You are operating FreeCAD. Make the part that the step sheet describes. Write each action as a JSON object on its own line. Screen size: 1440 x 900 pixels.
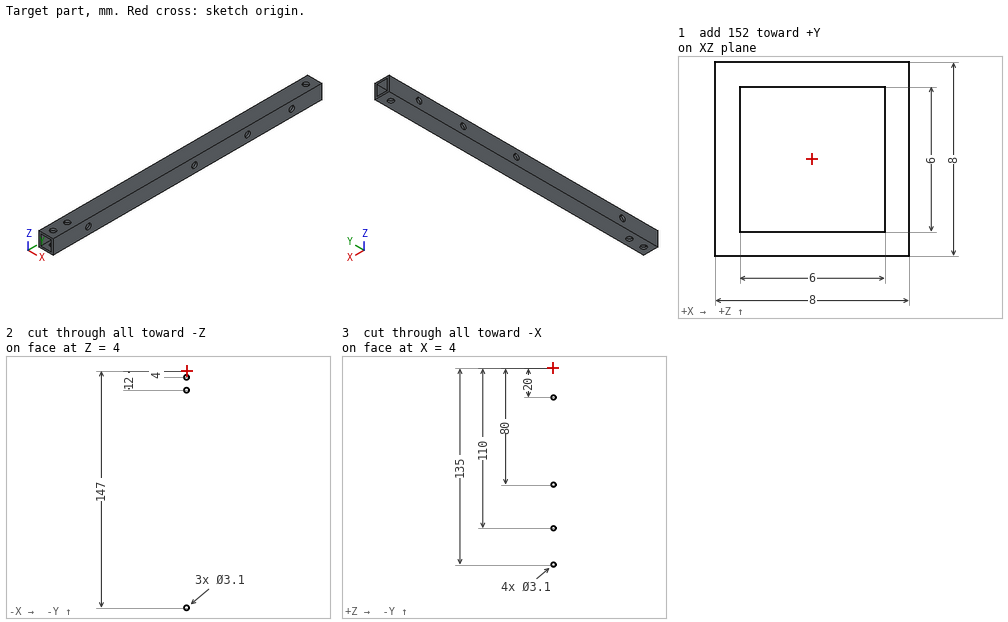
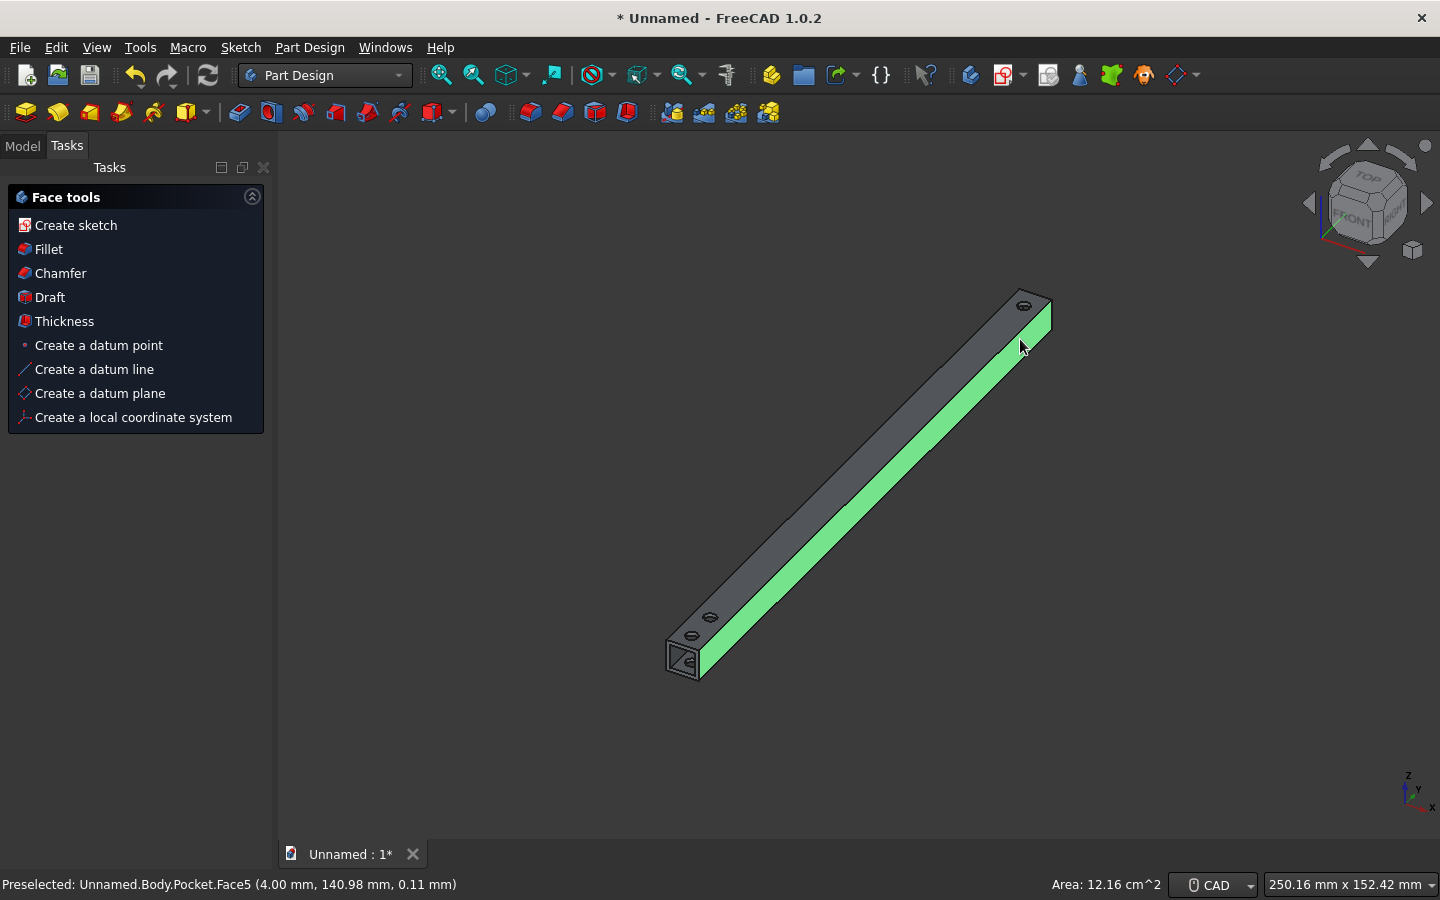
{"action": "left_click", "coordinate": [1004, 76]}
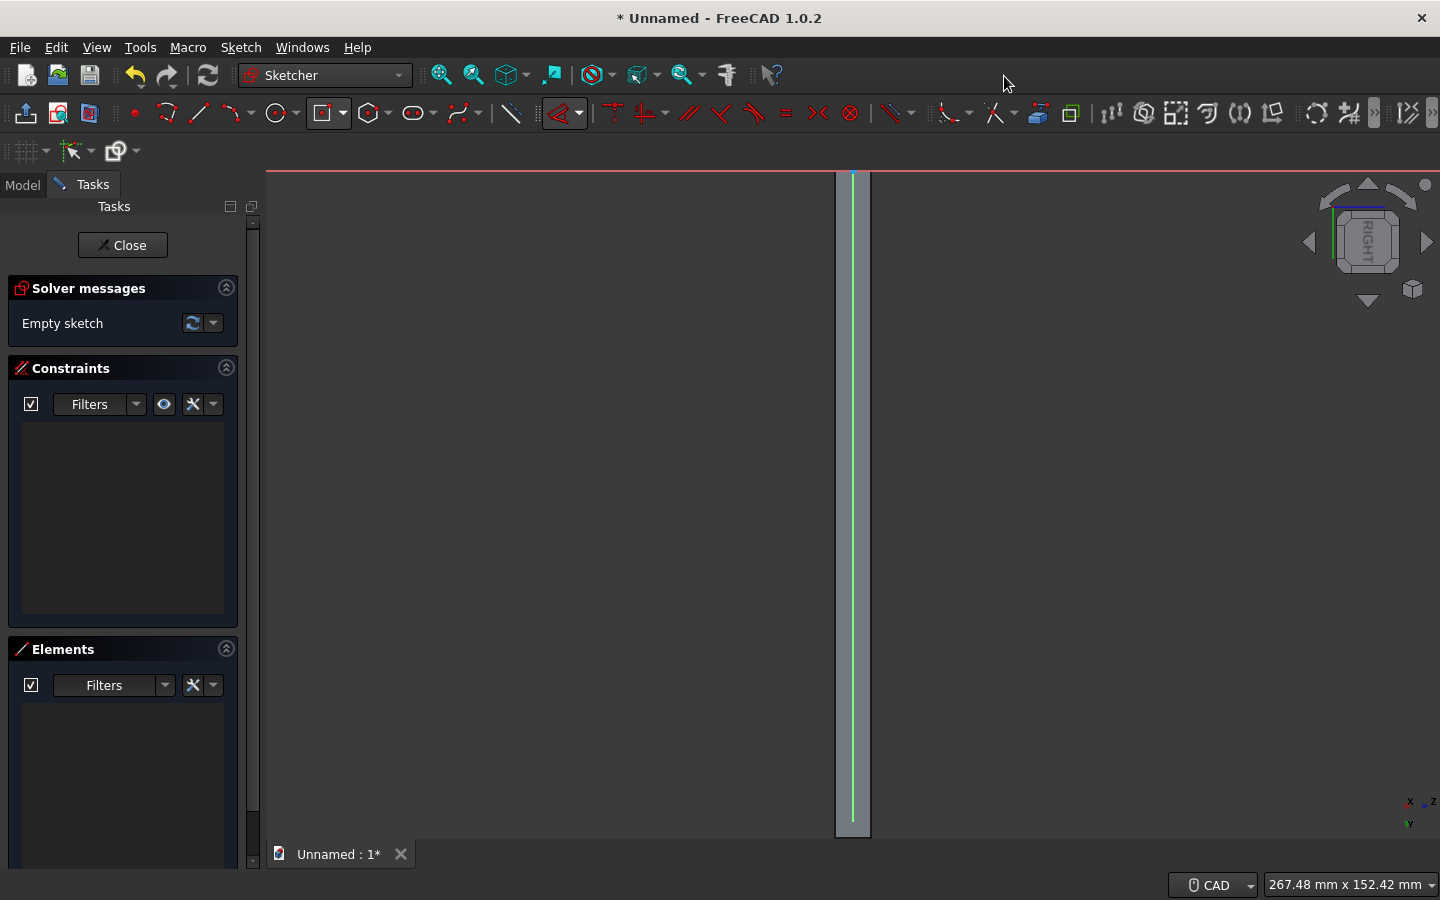
{"action": "scroll", "coordinate": [645, 573], "scroll_direction": "down", "scroll_amount": 2}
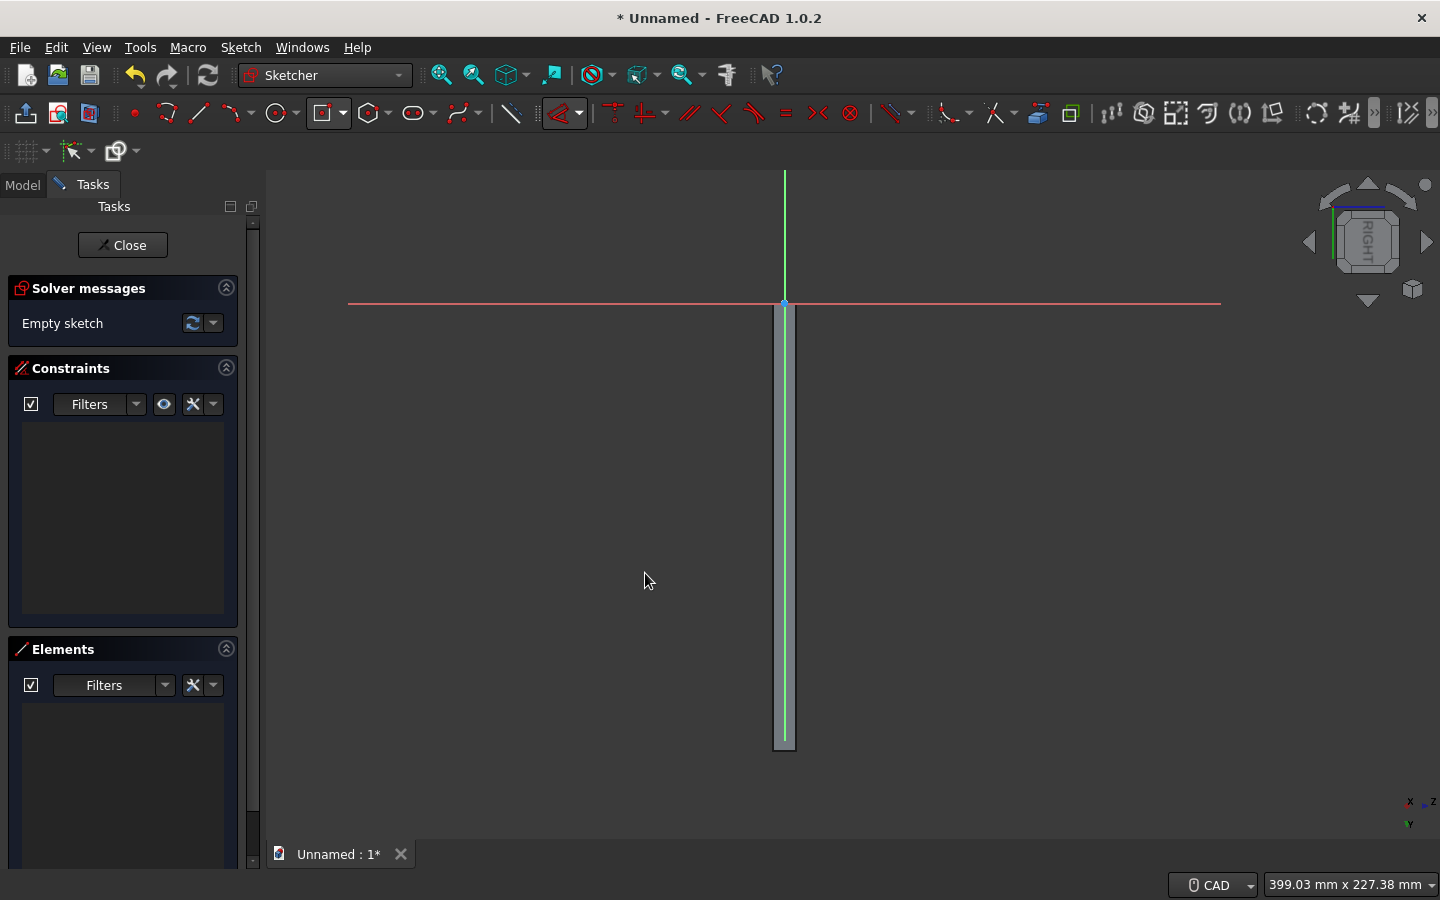
{"action": "key", "text": "g c"}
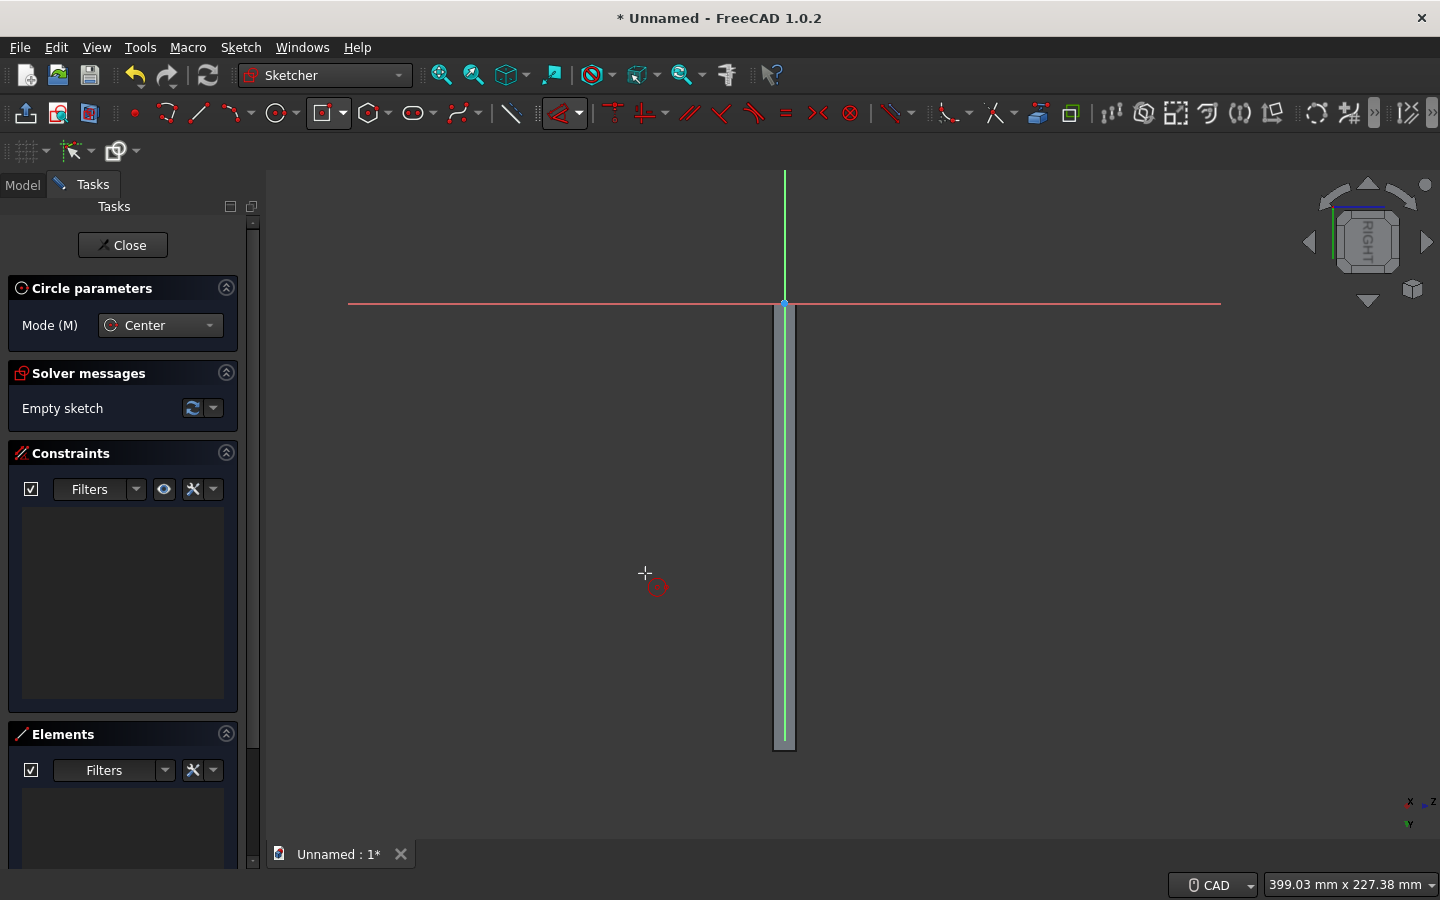
{"action": "scroll", "coordinate": [785, 701], "scroll_direction": "up", "scroll_amount": 9}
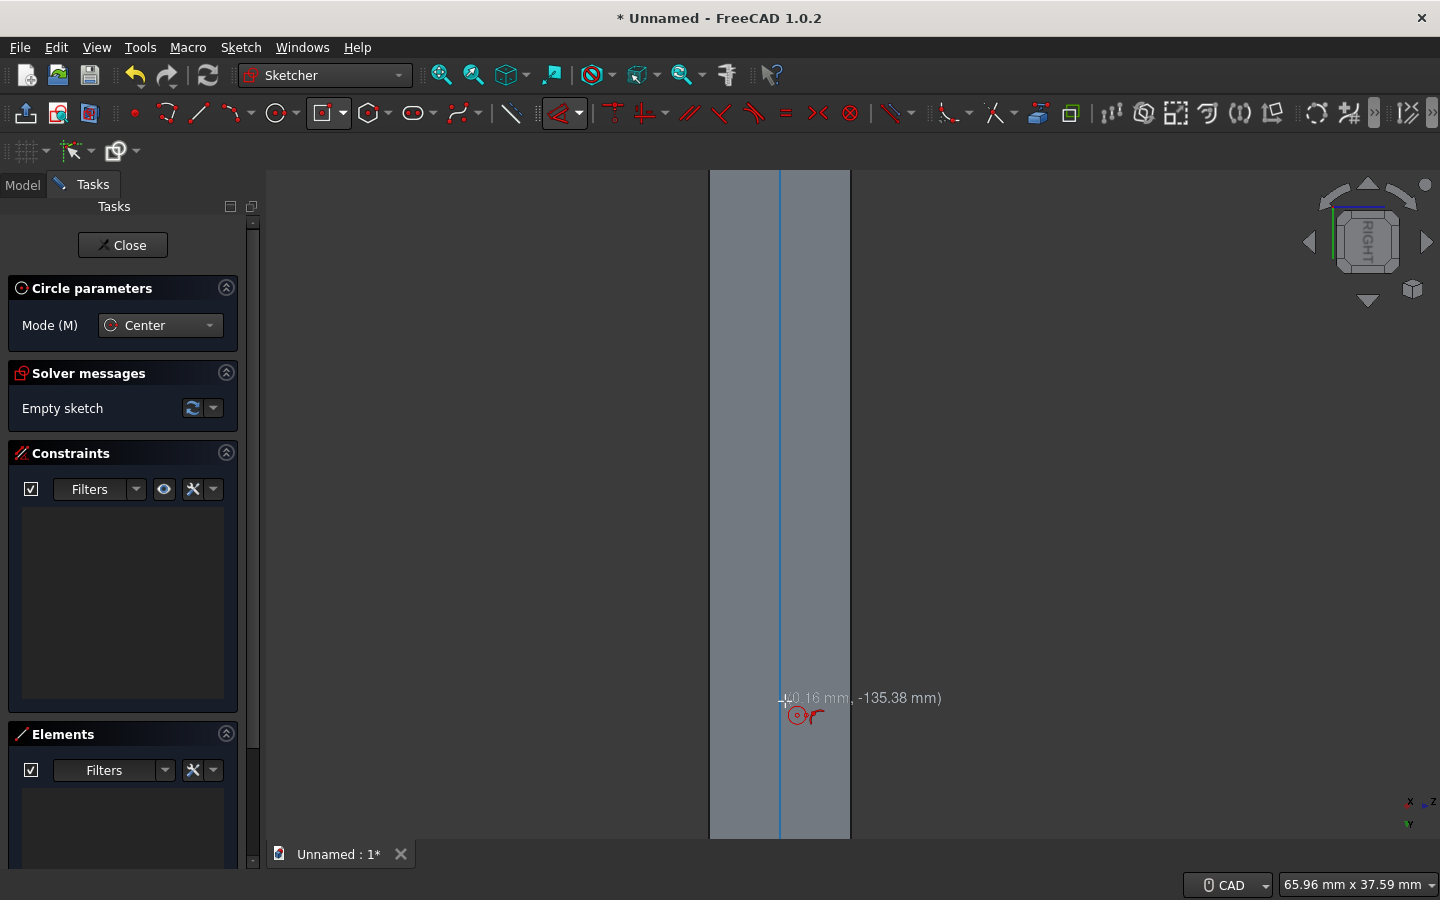
{"action": "scroll", "coordinate": [785, 702], "scroll_direction": "down", "scroll_amount": 9}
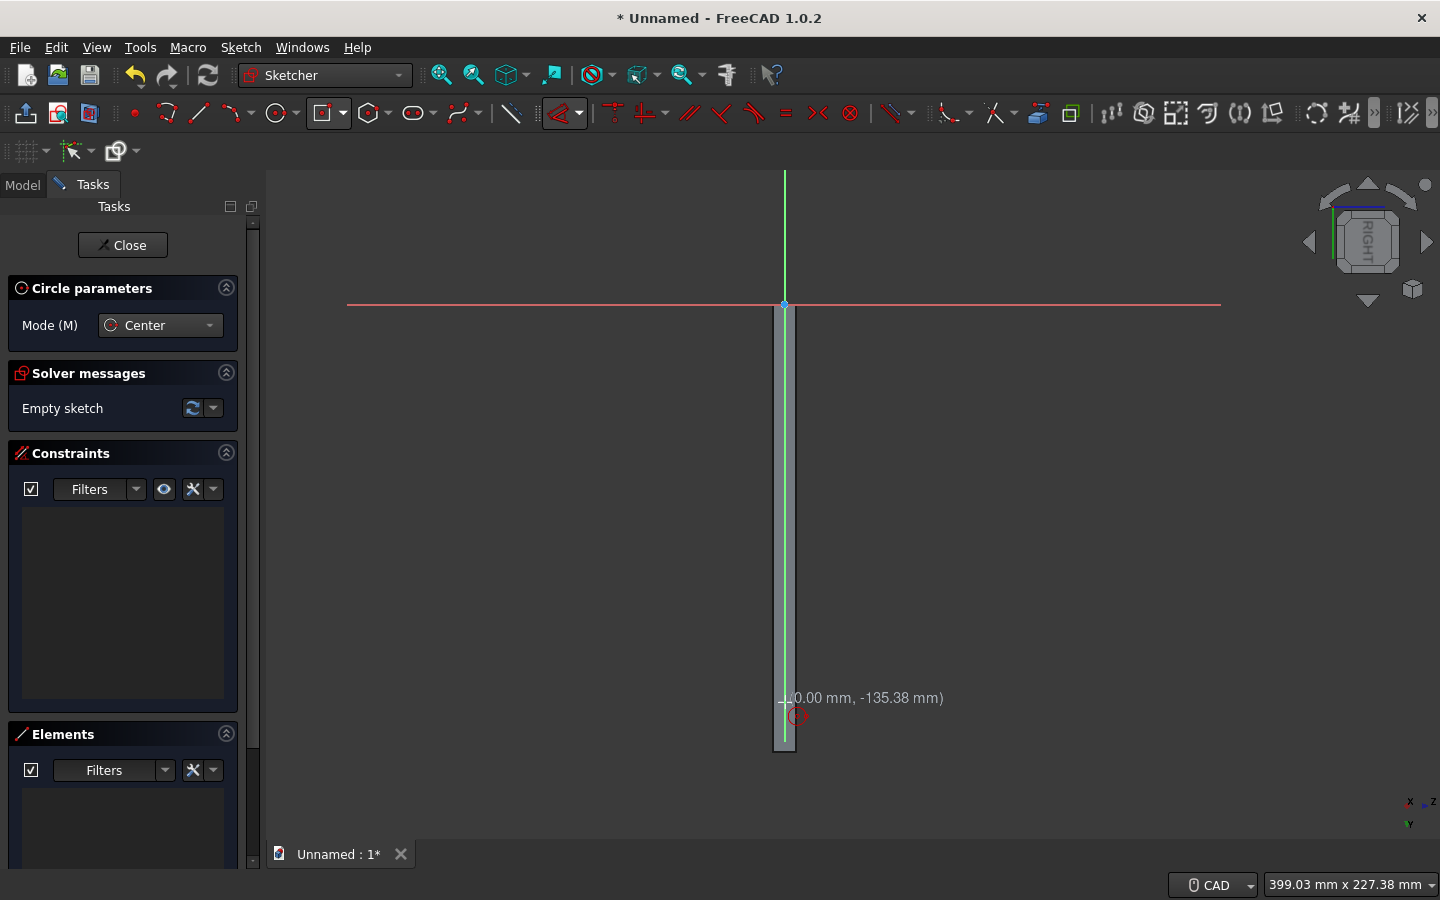
{"action": "left_click", "coordinate": [785, 702]}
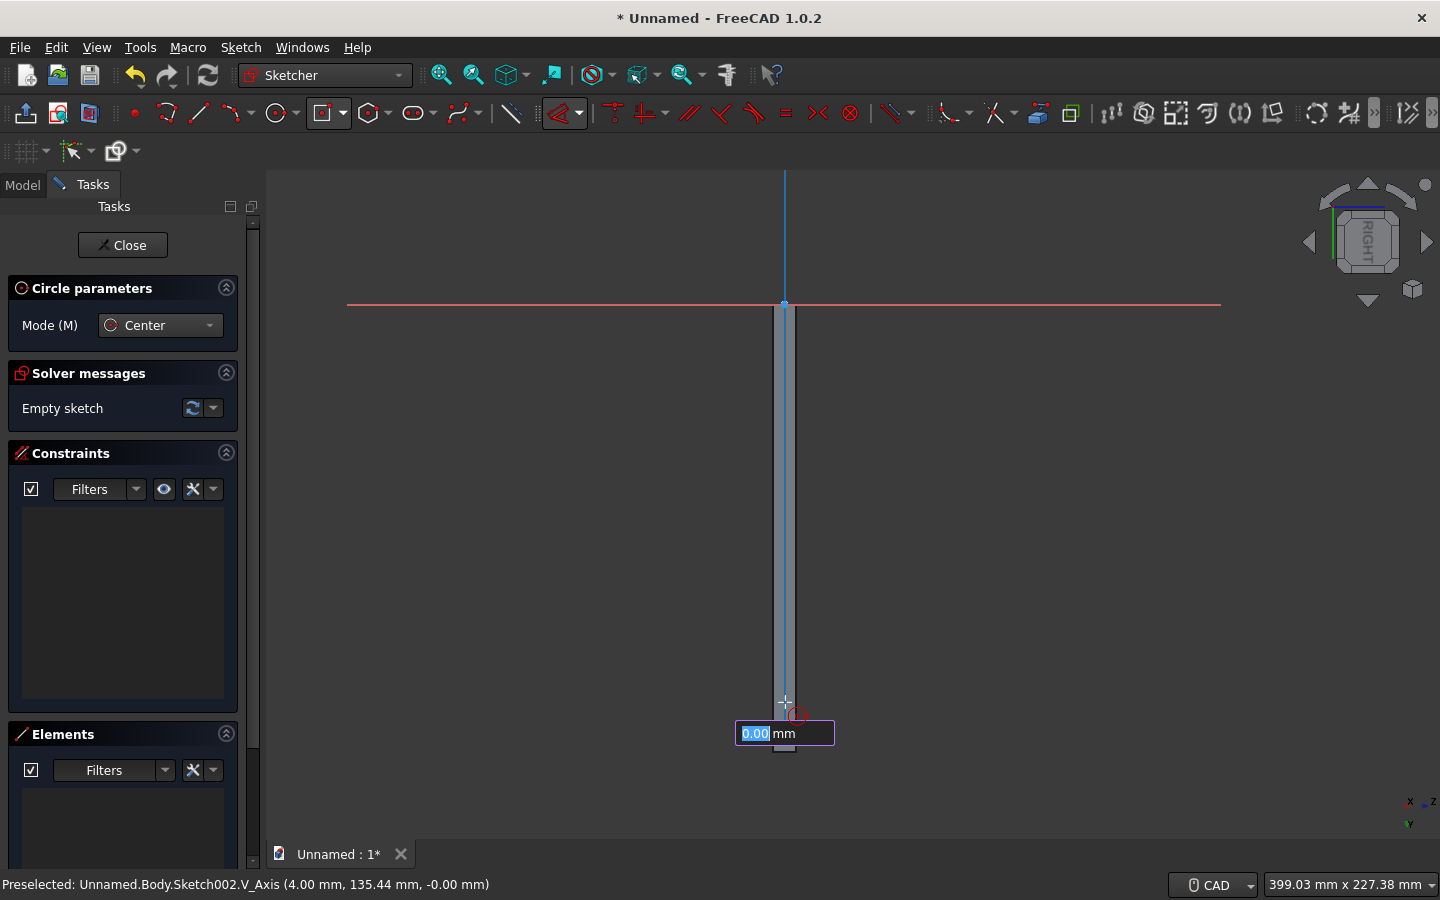
{"action": "scroll", "coordinate": [789, 700], "scroll_direction": "up", "scroll_amount": 7}
{"action": "mouse_move", "coordinate": [787, 698]}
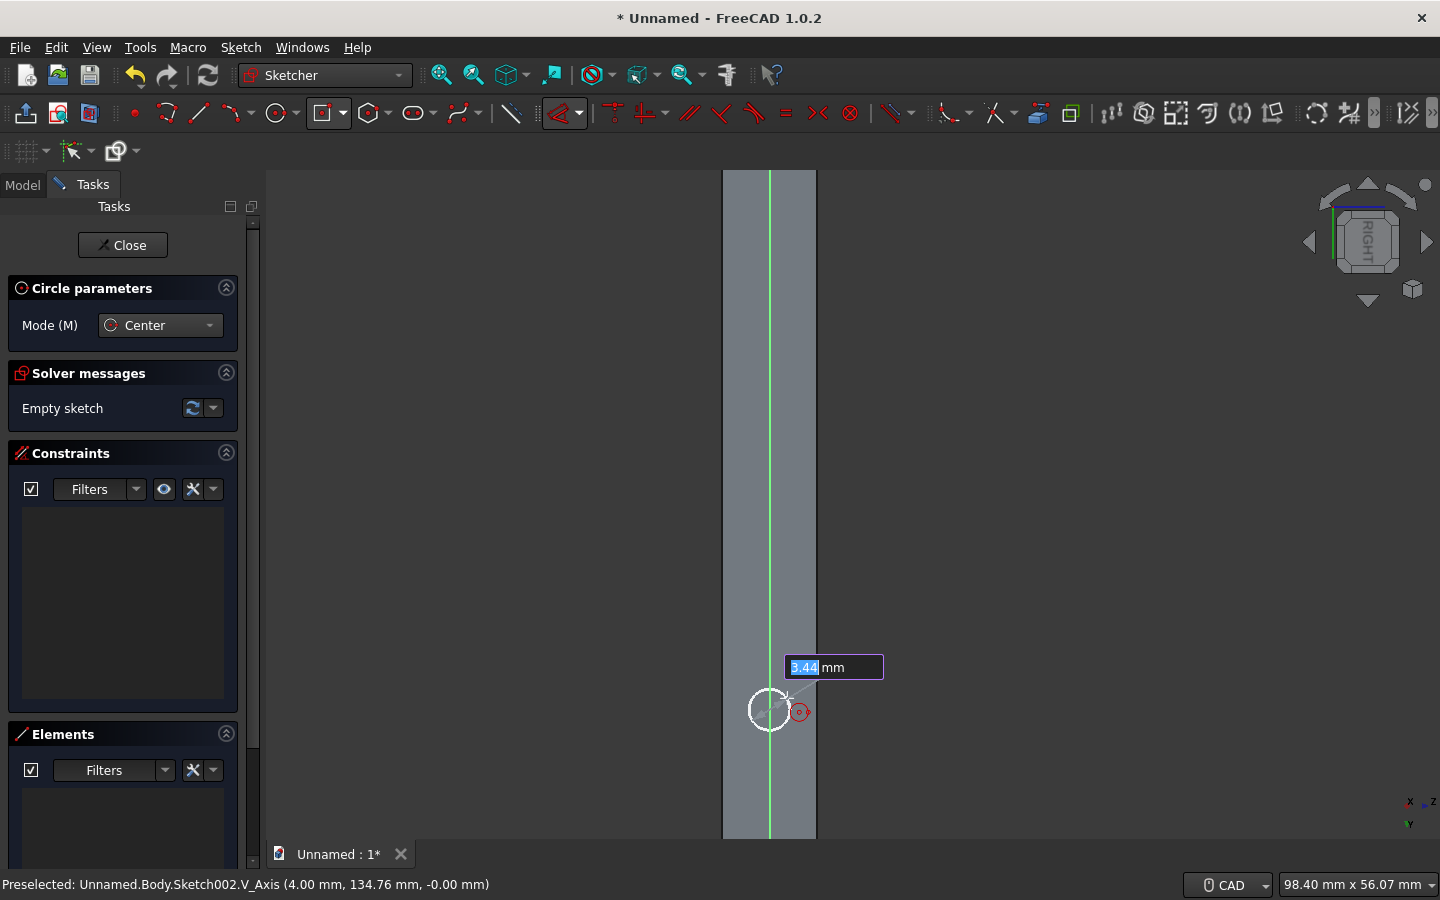
{"action": "type", "text": "3.1"}
{"action": "key", "text": "Return"}